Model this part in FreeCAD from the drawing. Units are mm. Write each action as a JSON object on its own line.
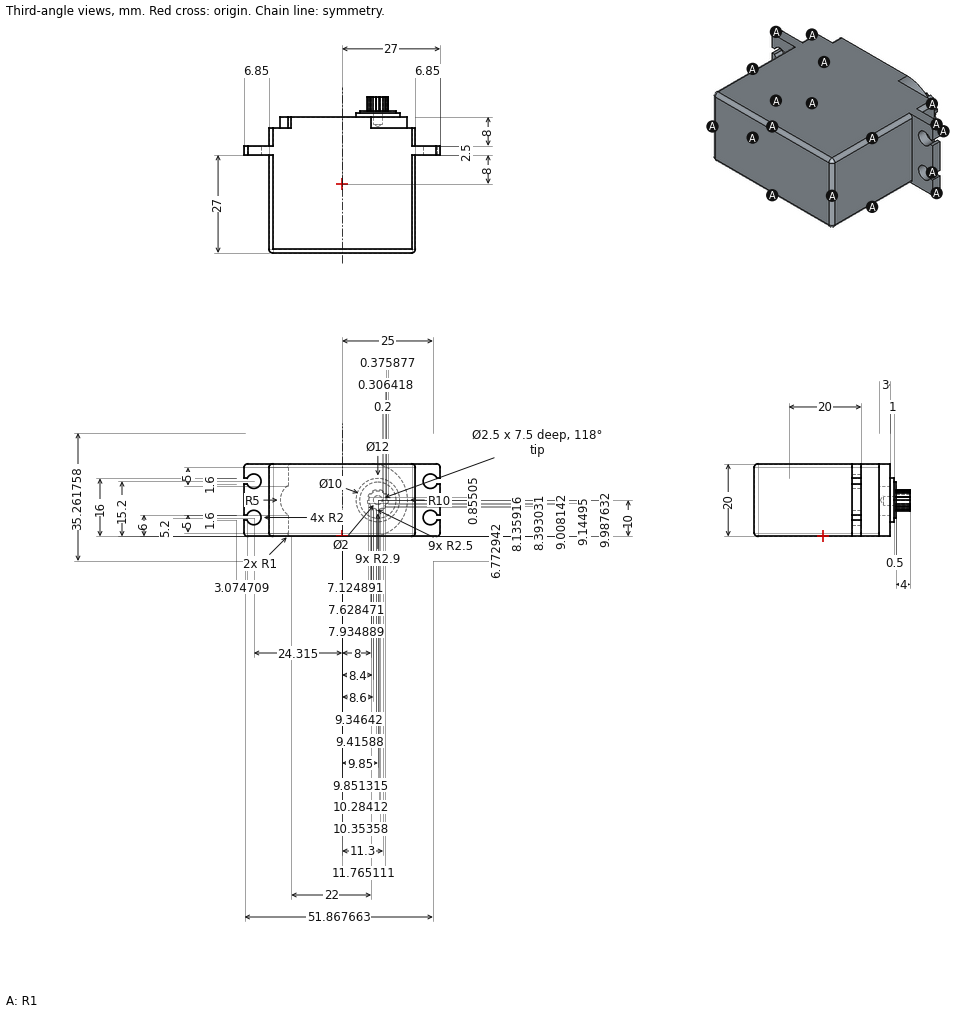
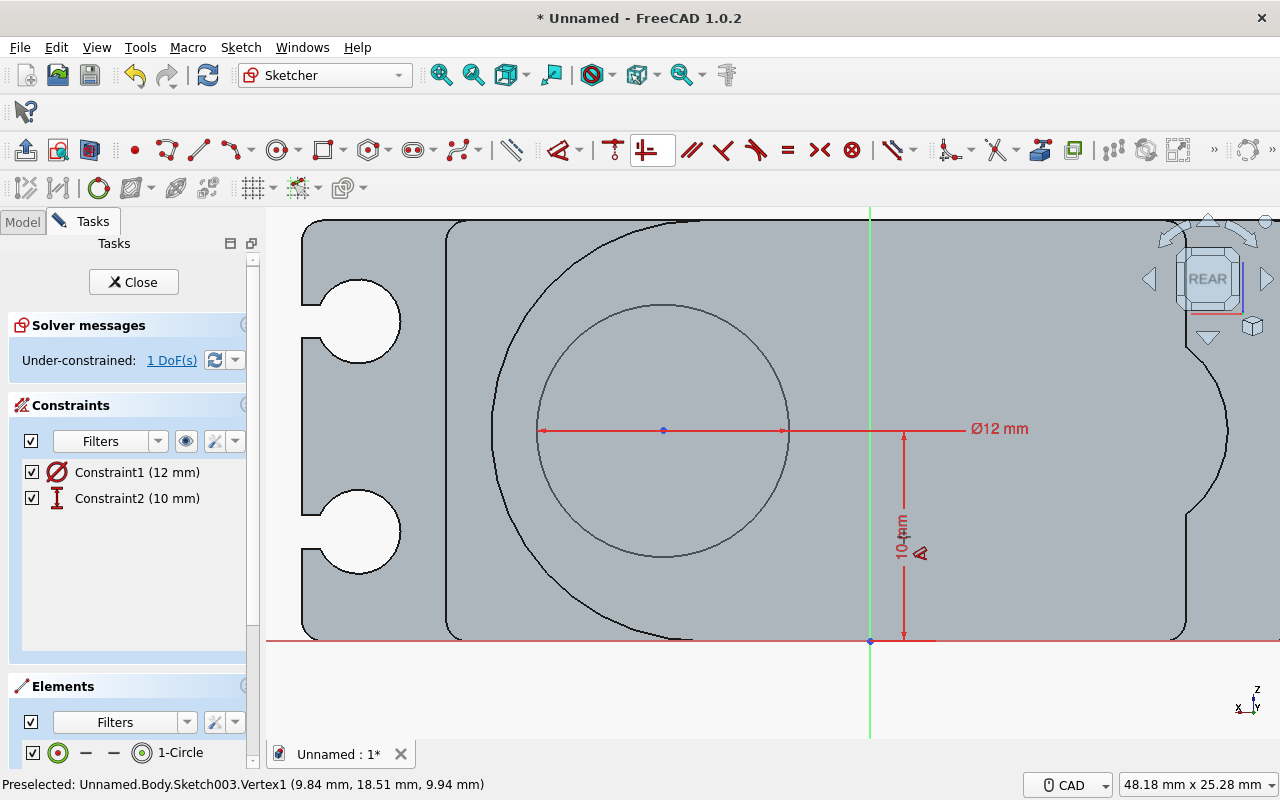
{"action": "left_click", "coordinate": [663, 431]}
{"action": "left_click", "coordinate": [767, 675]}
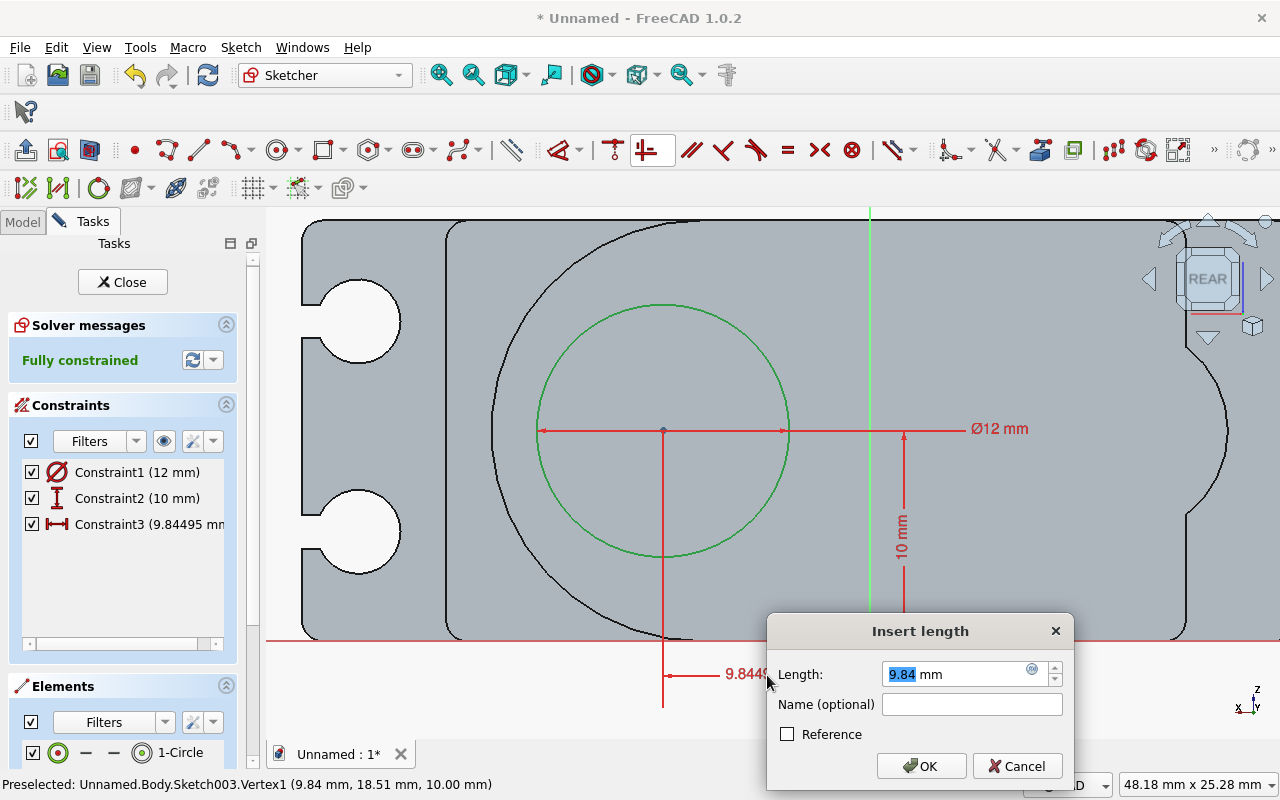
{"action": "type", "text": "9.85"}
{"action": "key", "text": "Return"}
{"action": "key", "text": "Escape"}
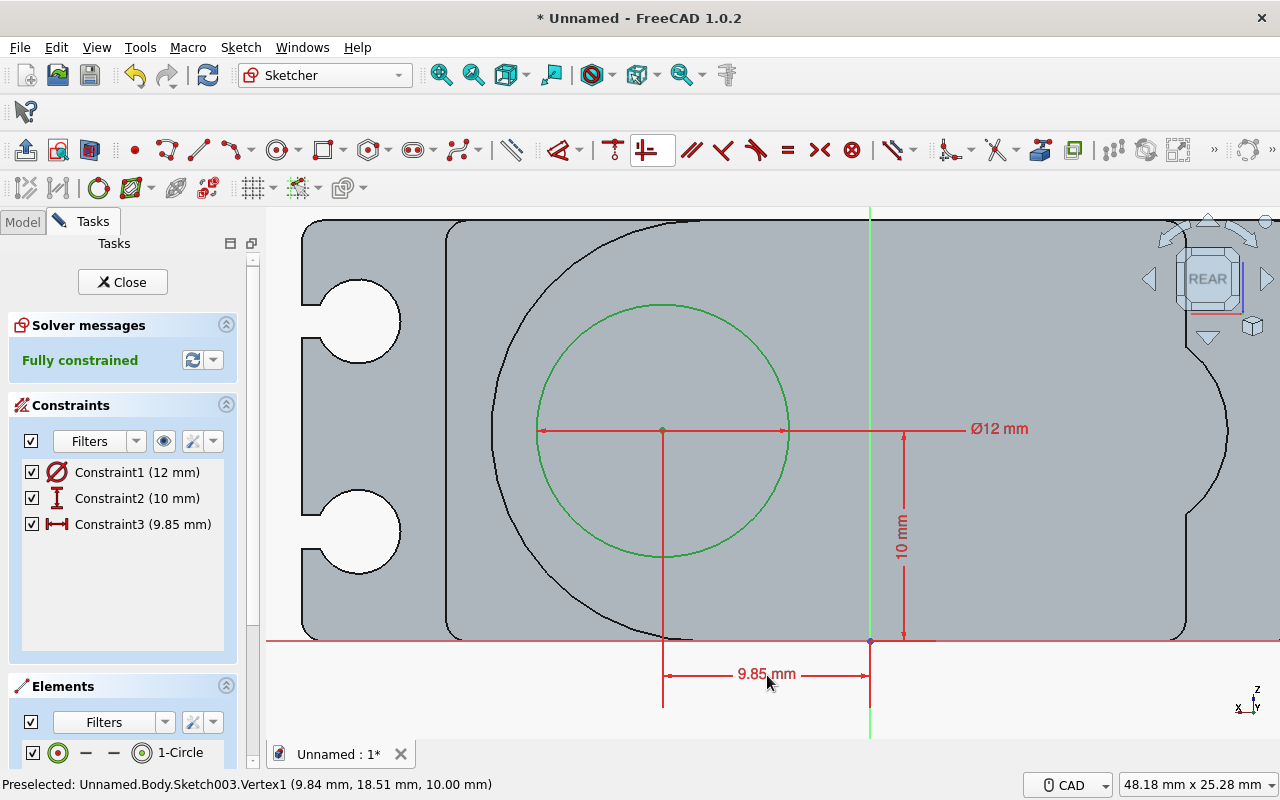
{"action": "left_click", "coordinate": [123, 282]}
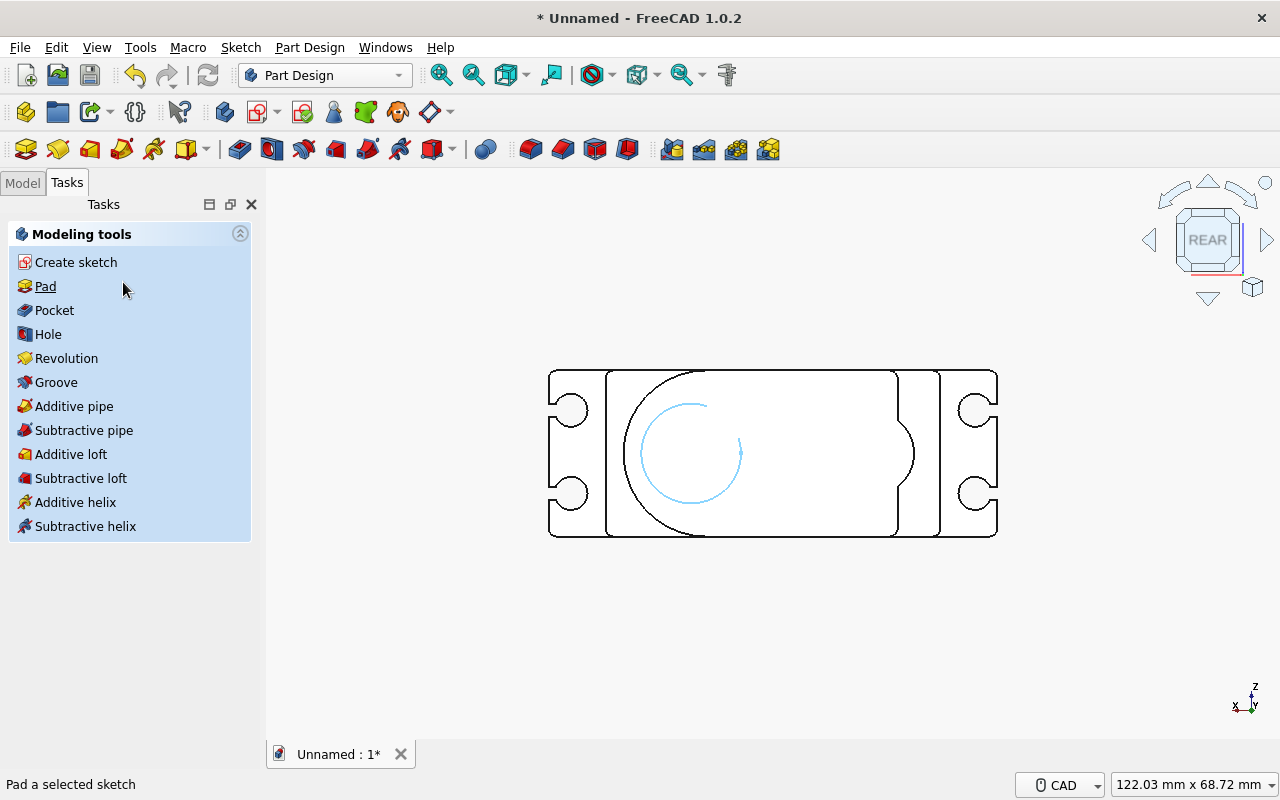
{"action": "left_click", "coordinate": [26, 150]}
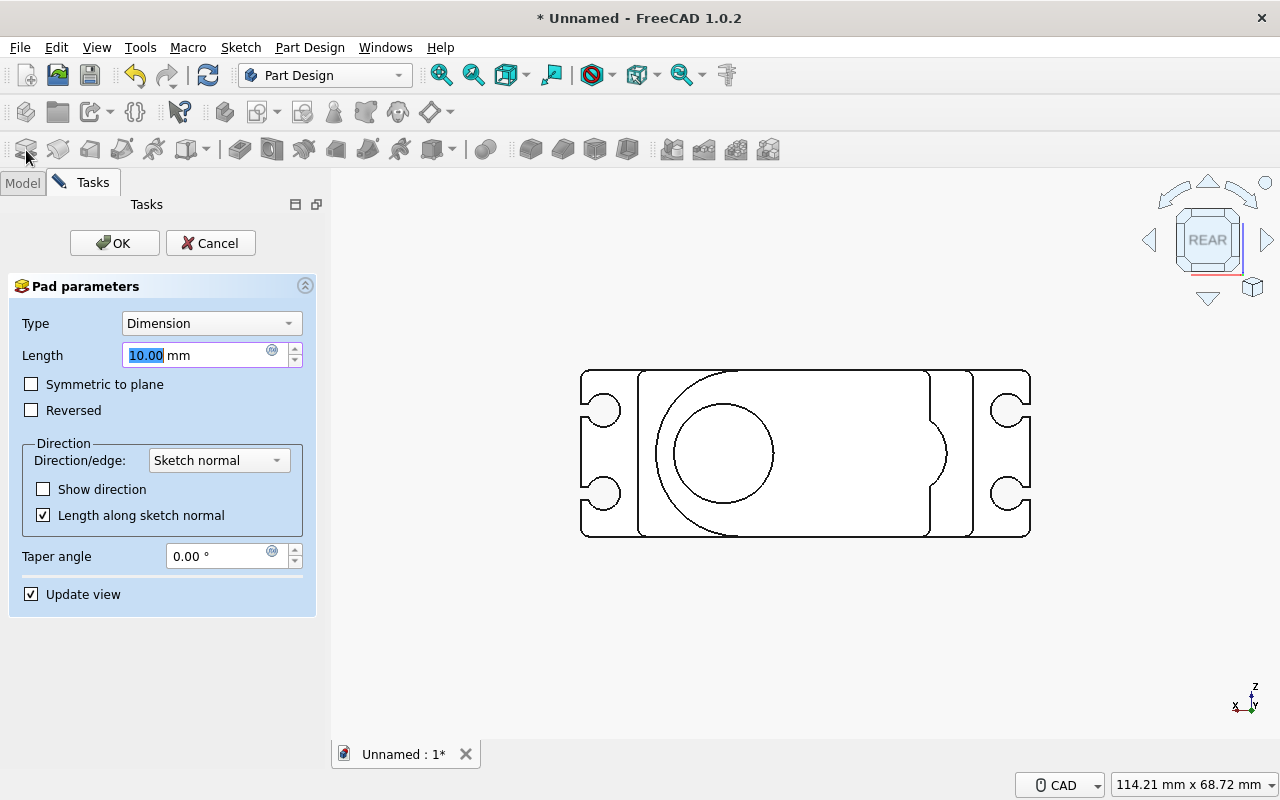
{"action": "type", "text": "1"}
{"action": "key", "text": "Tab"}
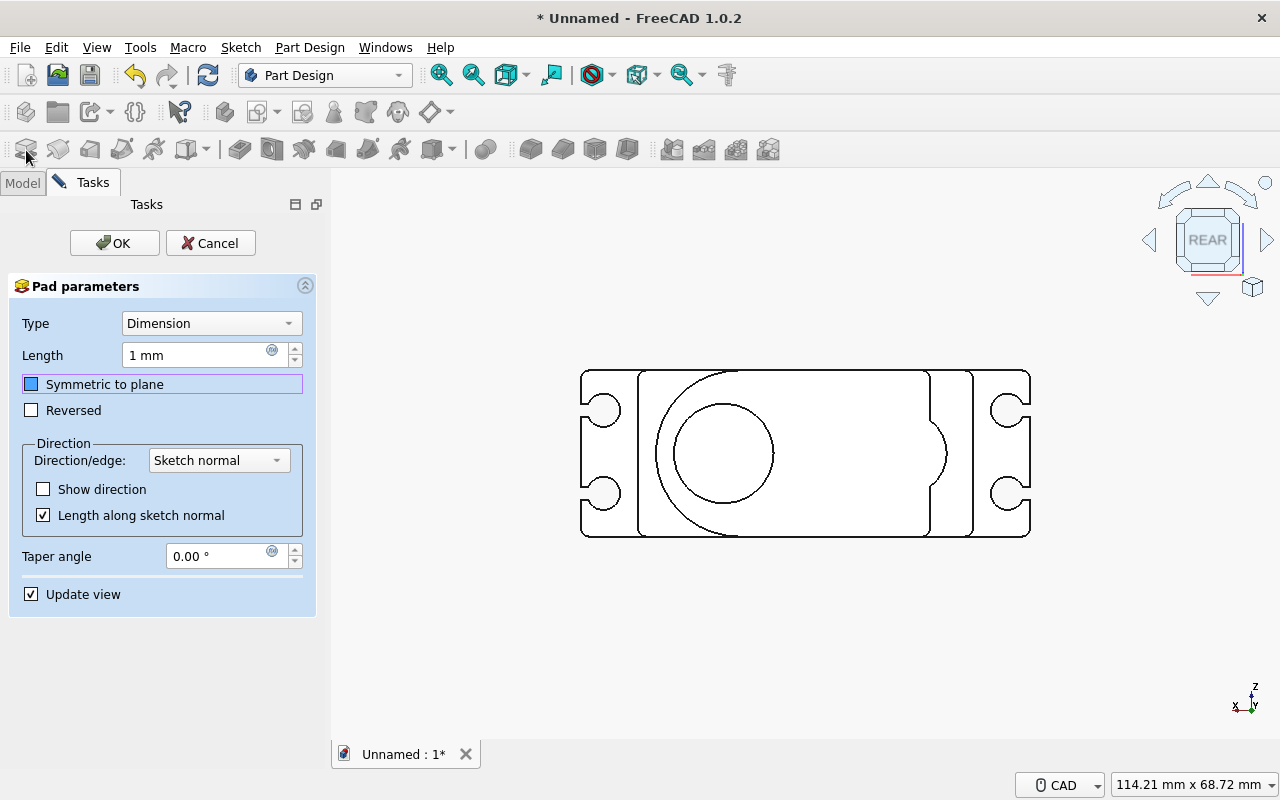
{"action": "left_click", "coordinate": [115, 243]}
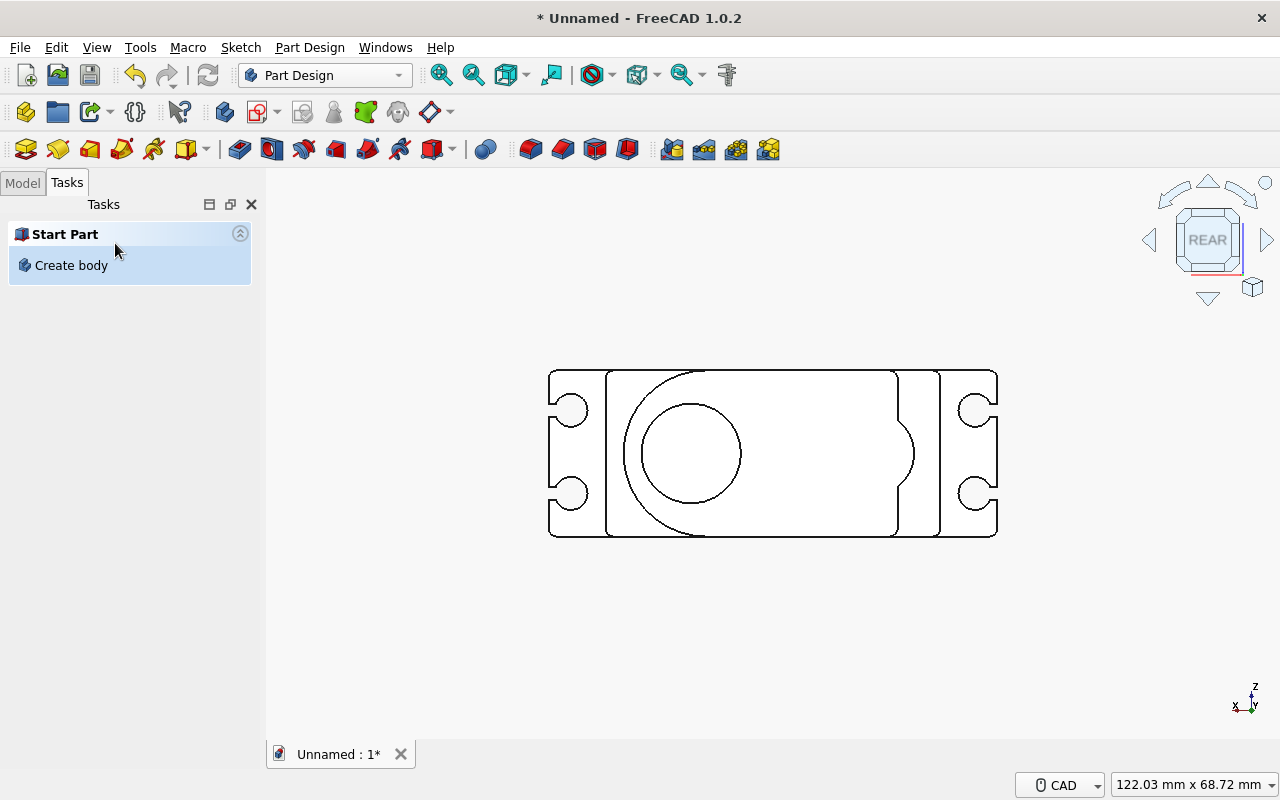
{"action": "key", "text": "v f"}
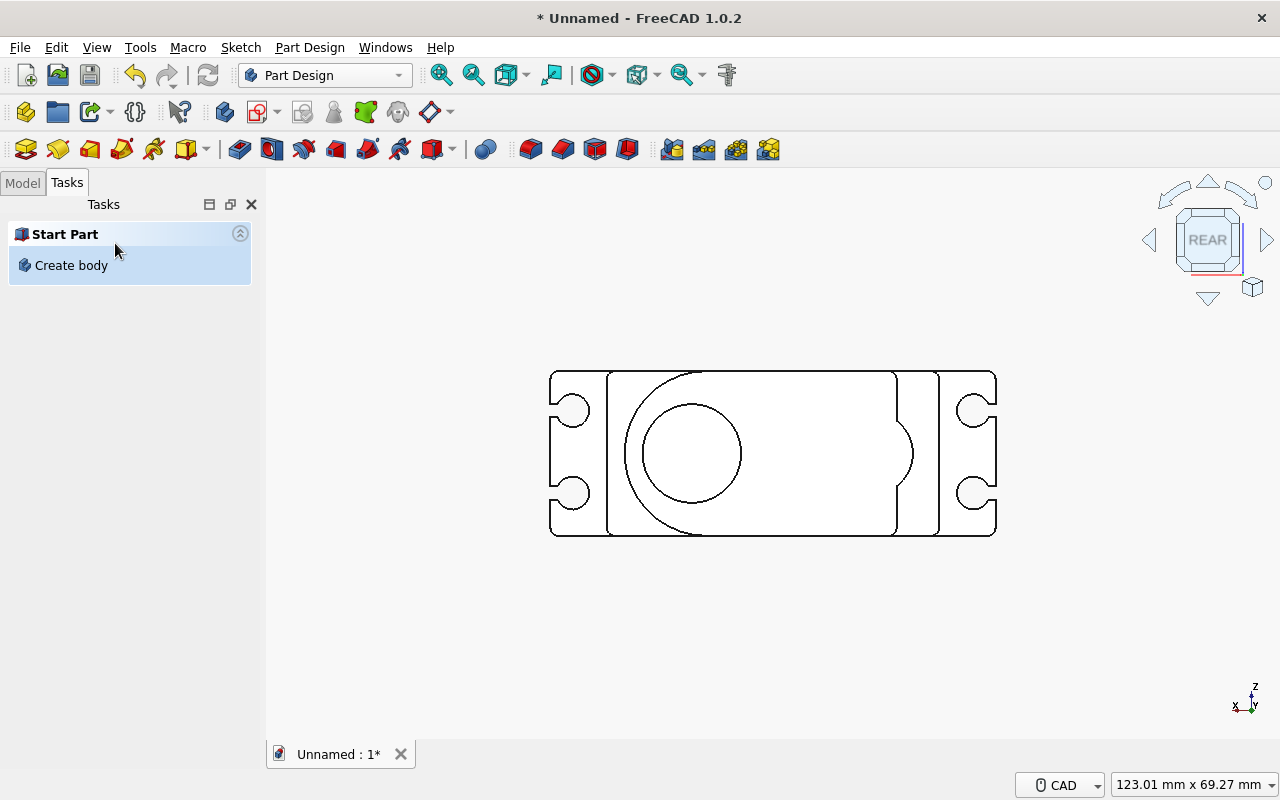
{"action": "left_click", "coordinate": [692, 452]}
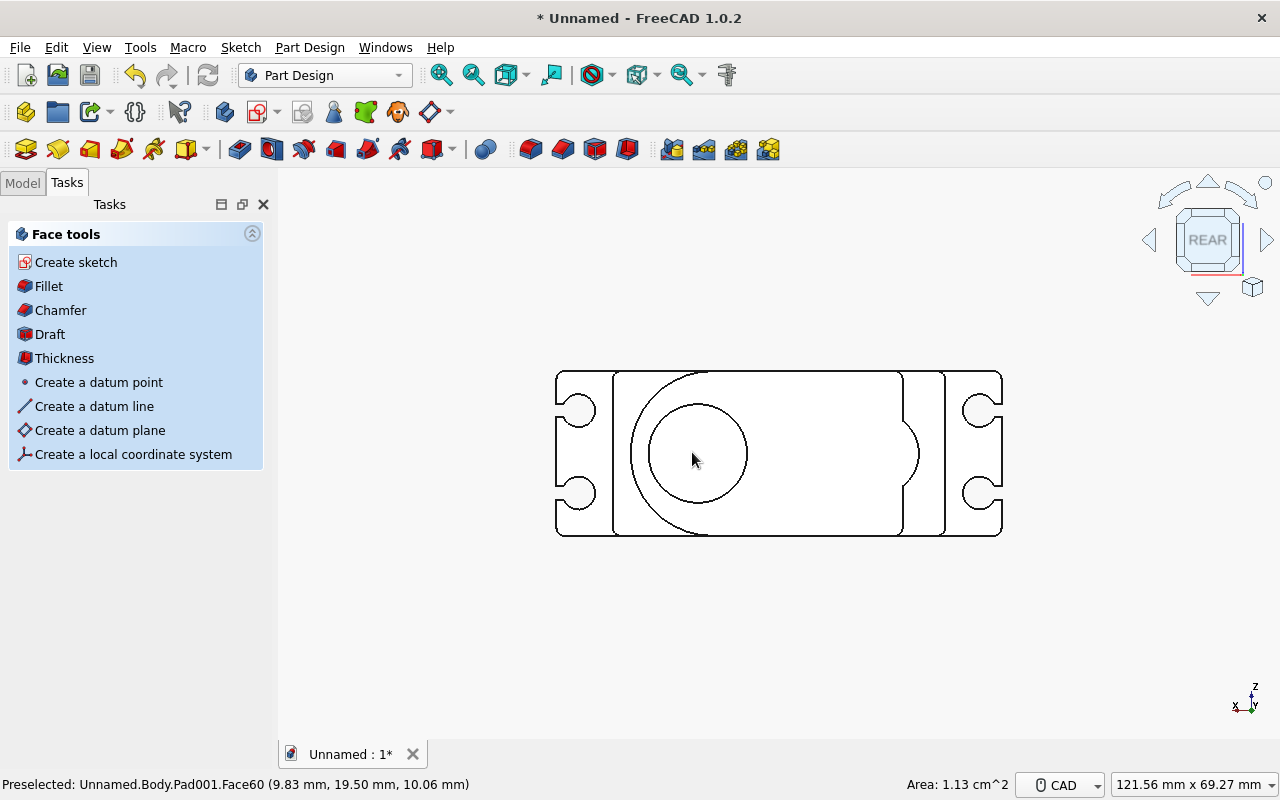
{"action": "left_click", "coordinate": [258, 112]}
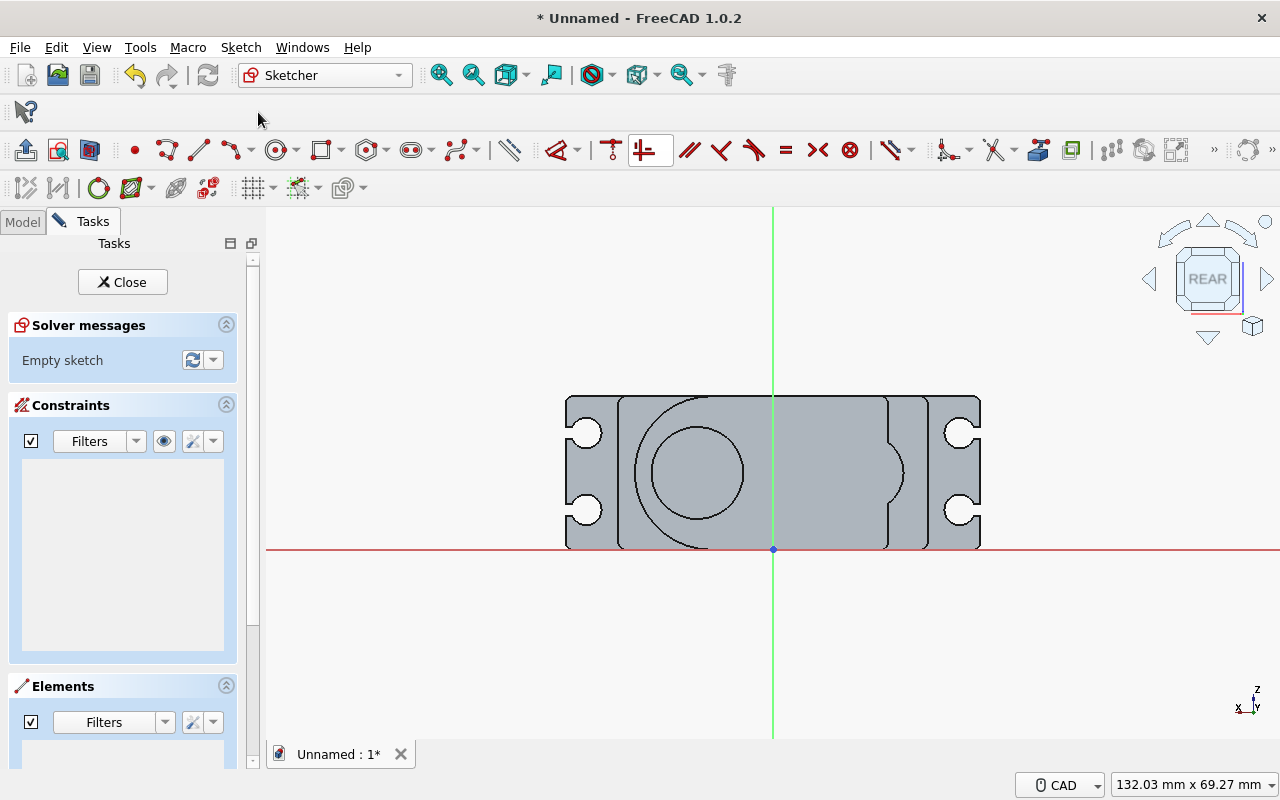
{"action": "scroll", "coordinate": [723, 503], "scroll_direction": "up", "scroll_amount": 5}